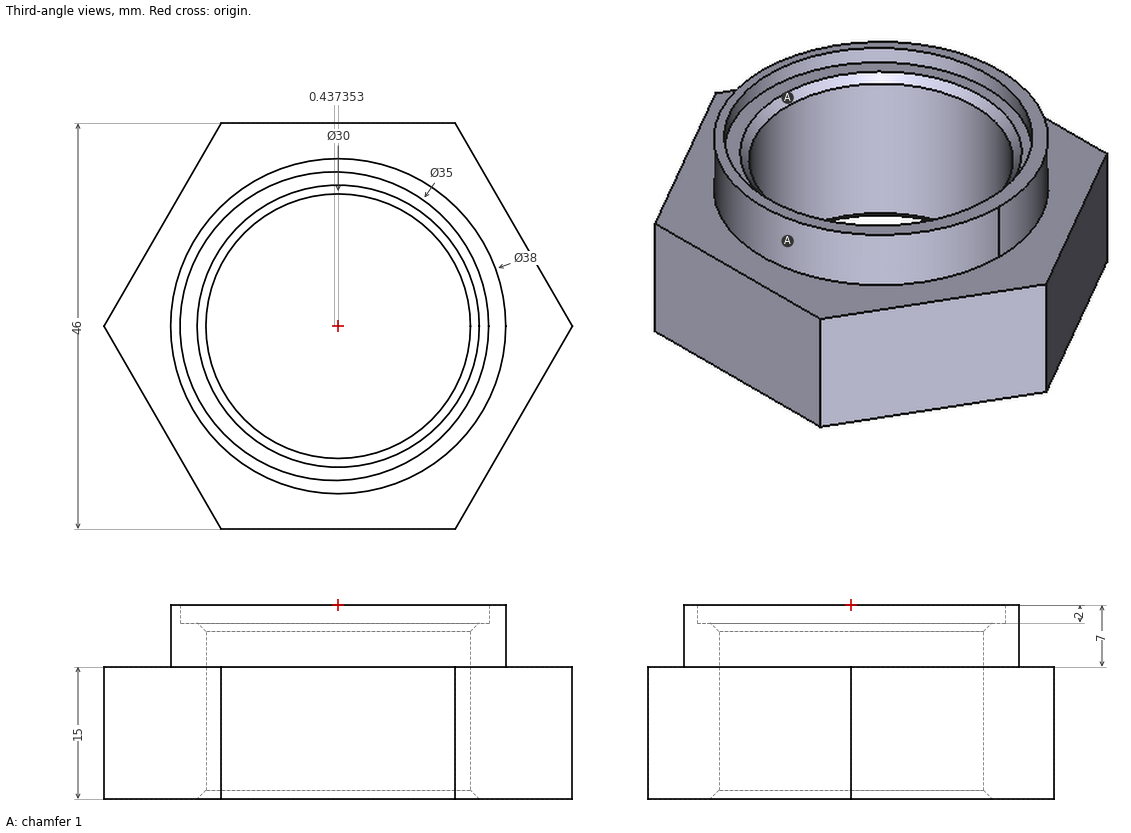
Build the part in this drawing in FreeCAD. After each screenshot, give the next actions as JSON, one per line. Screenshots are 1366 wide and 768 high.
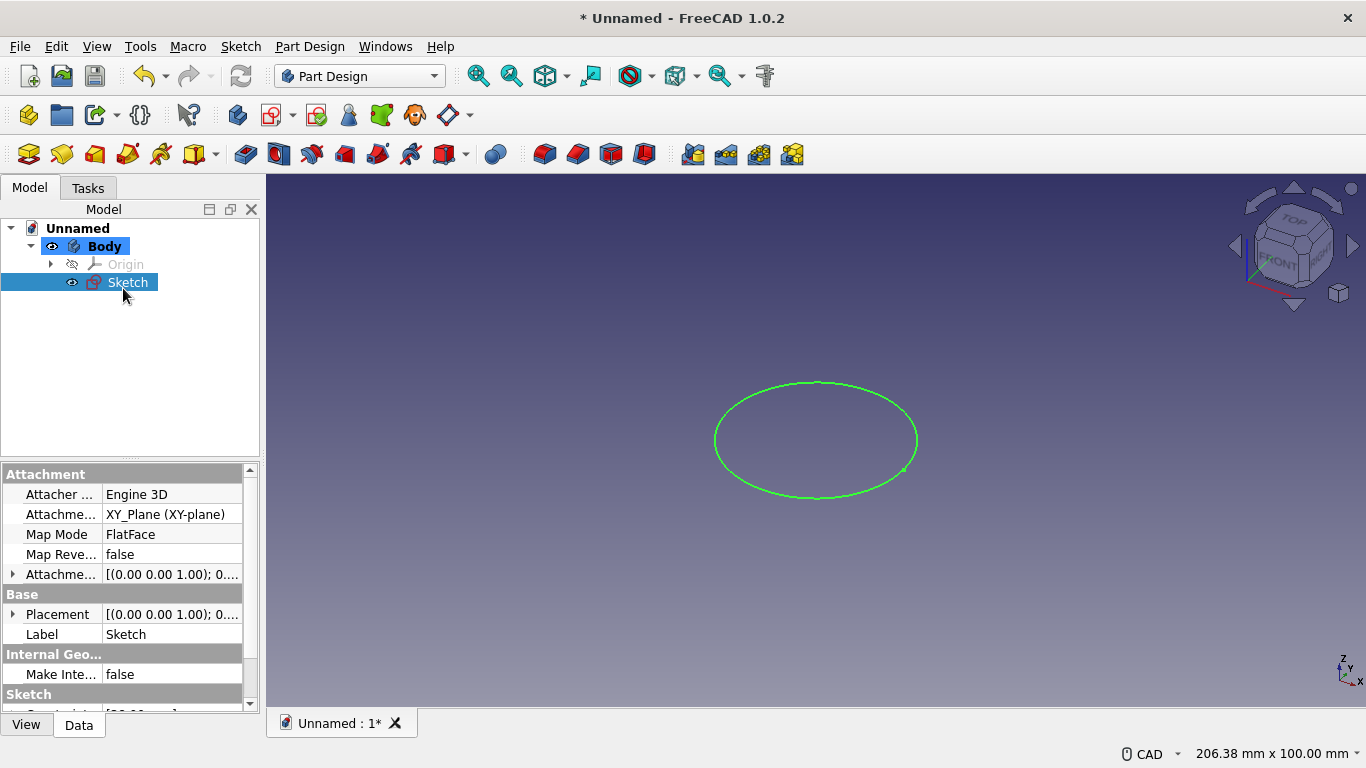
{"action": "left_click", "coordinate": [29, 154]}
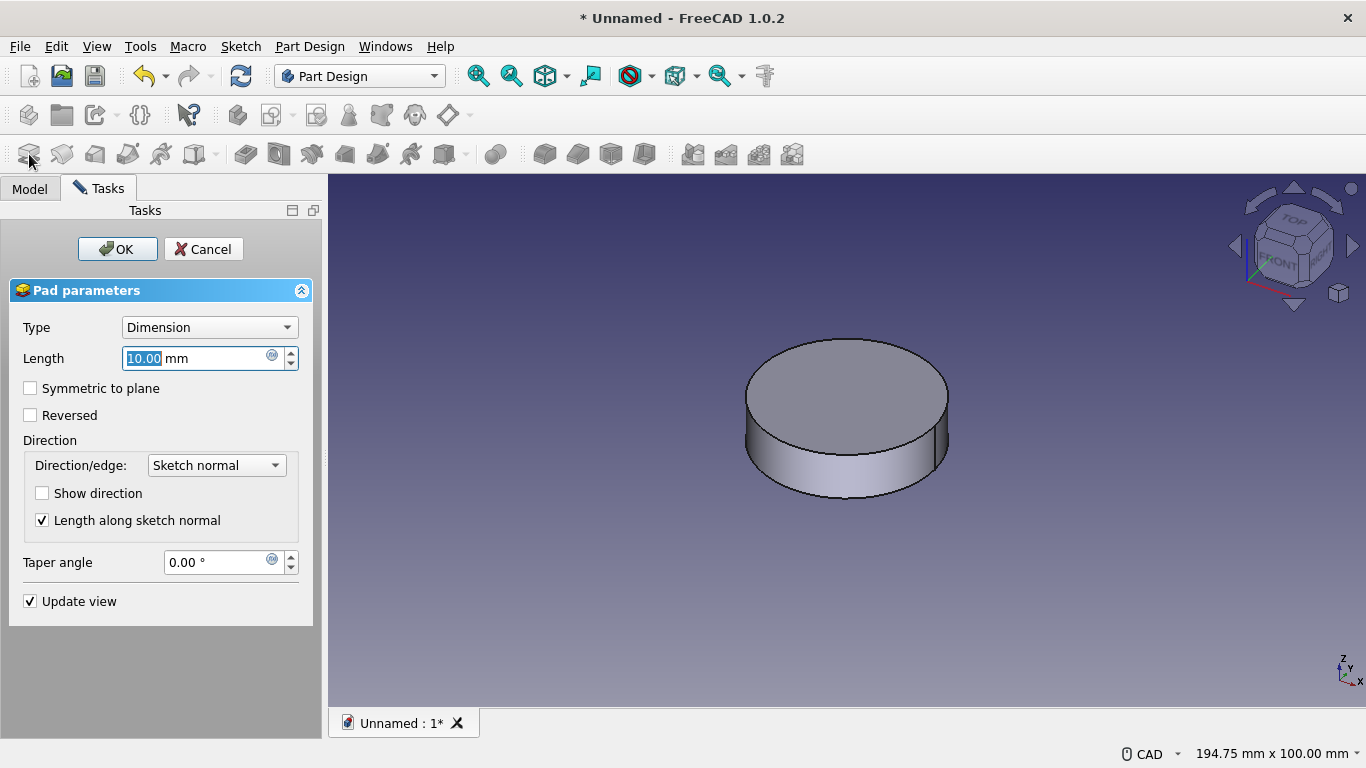
{"action": "type", "text": "7"}
{"action": "key", "text": "Tab"}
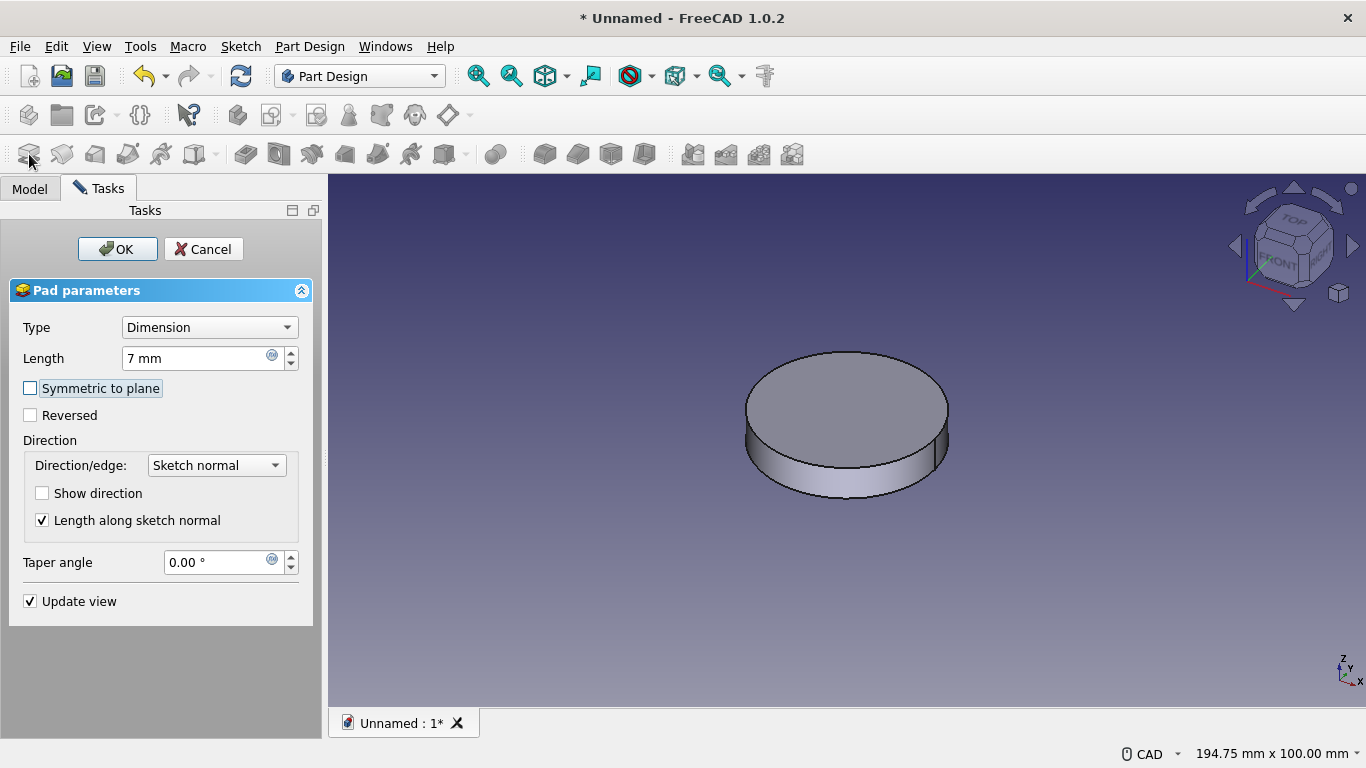
{"action": "left_click", "coordinate": [31, 415]}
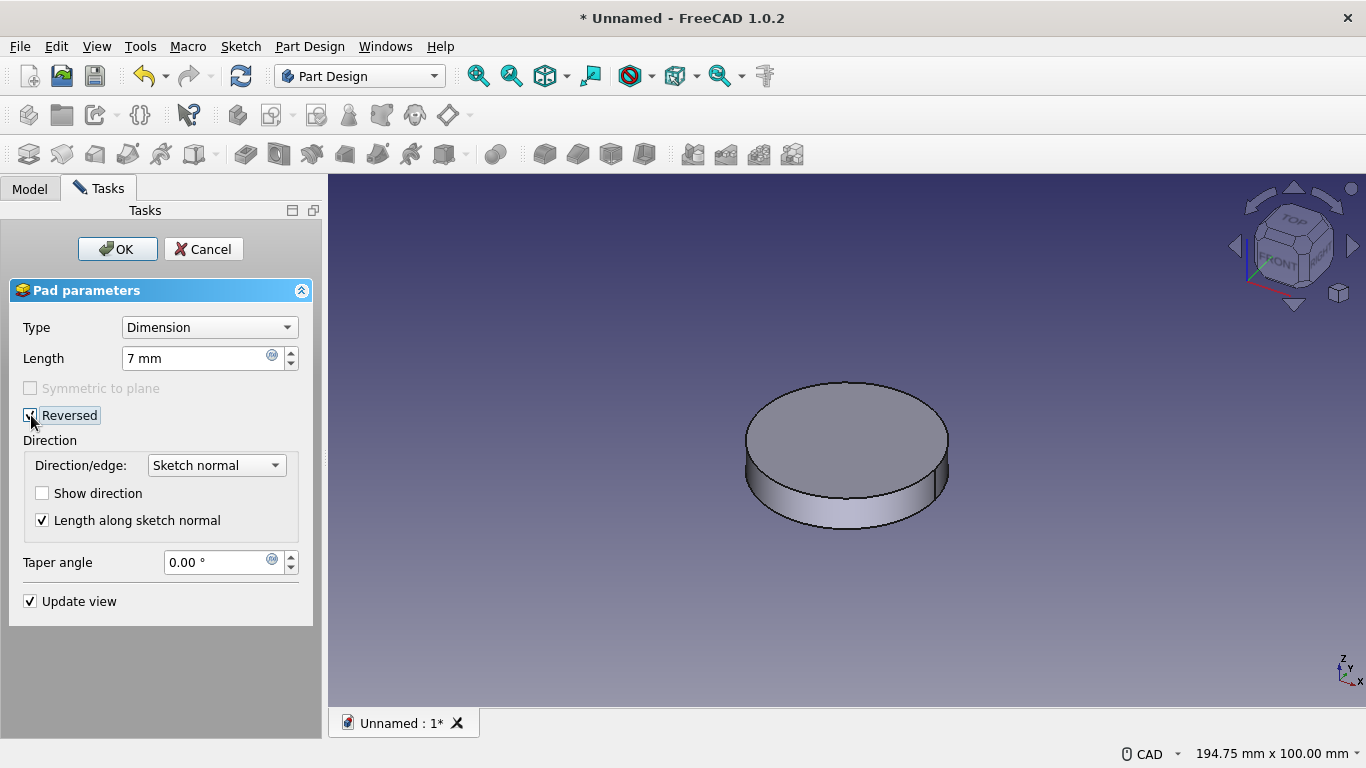
{"action": "left_click", "coordinate": [118, 249]}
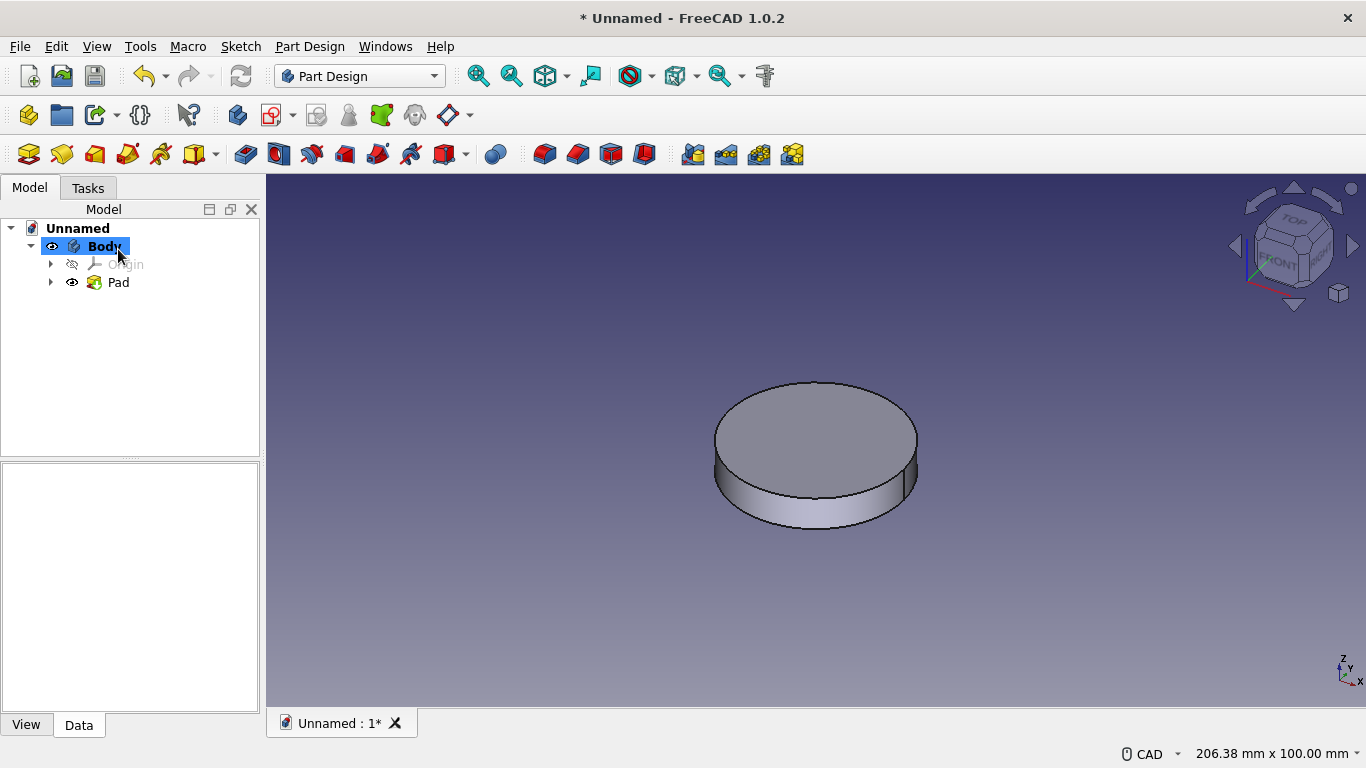
{"action": "left_click", "coordinate": [479, 76]}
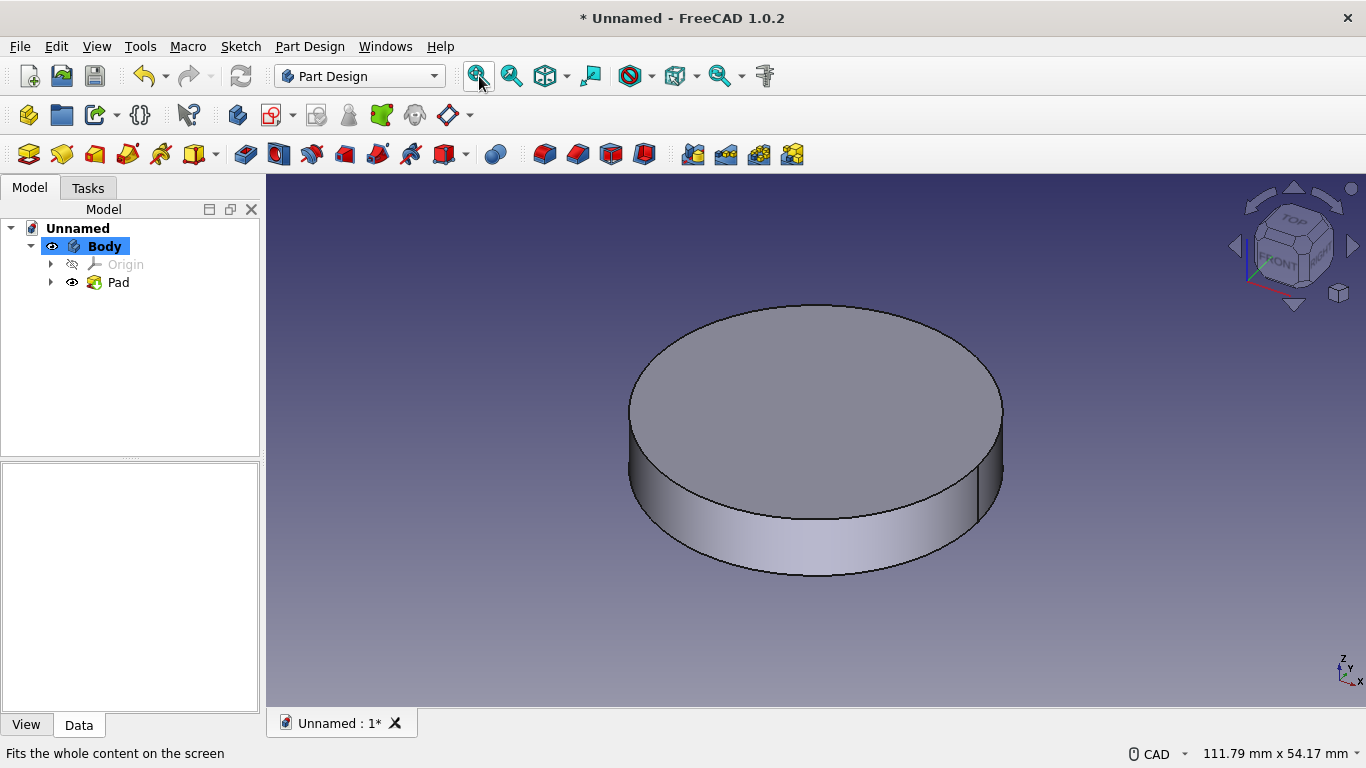
{"action": "key", "text": "5"}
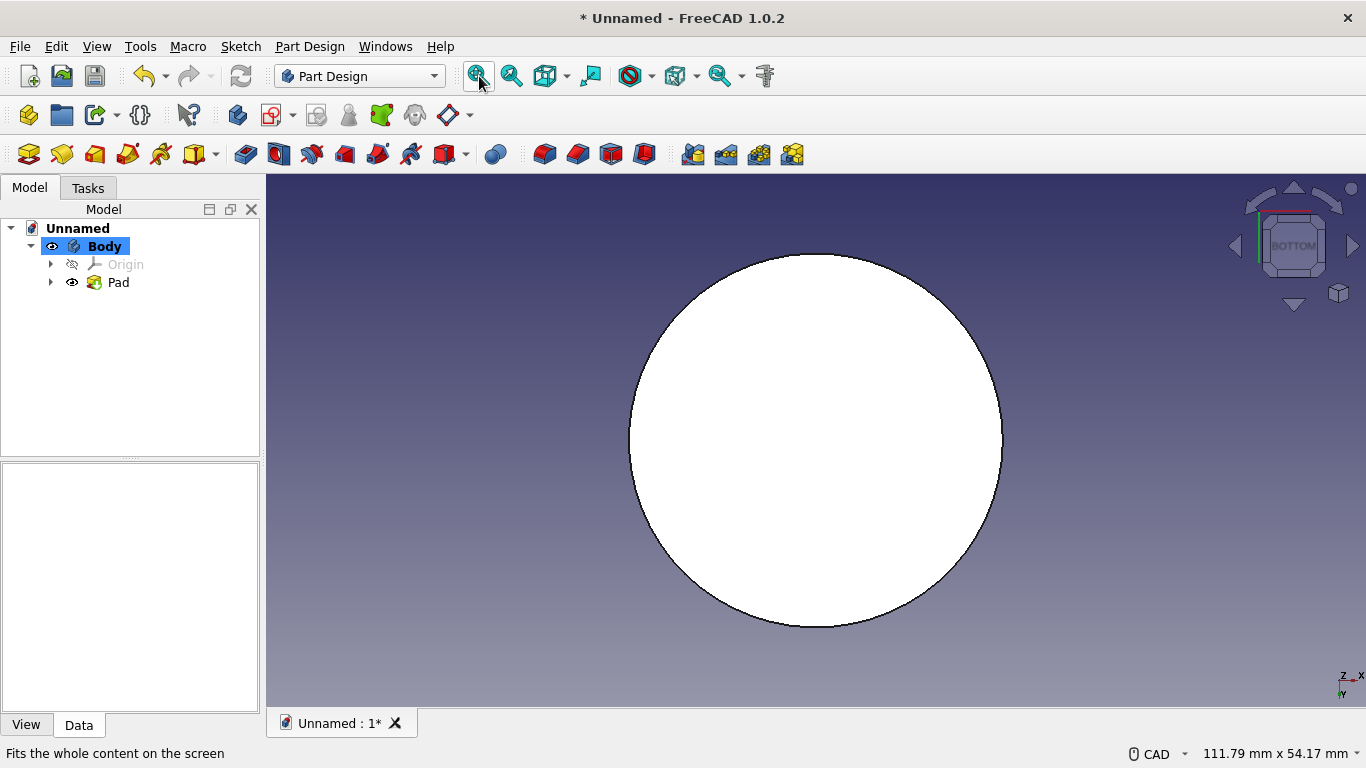
{"action": "left_click", "coordinate": [816, 439]}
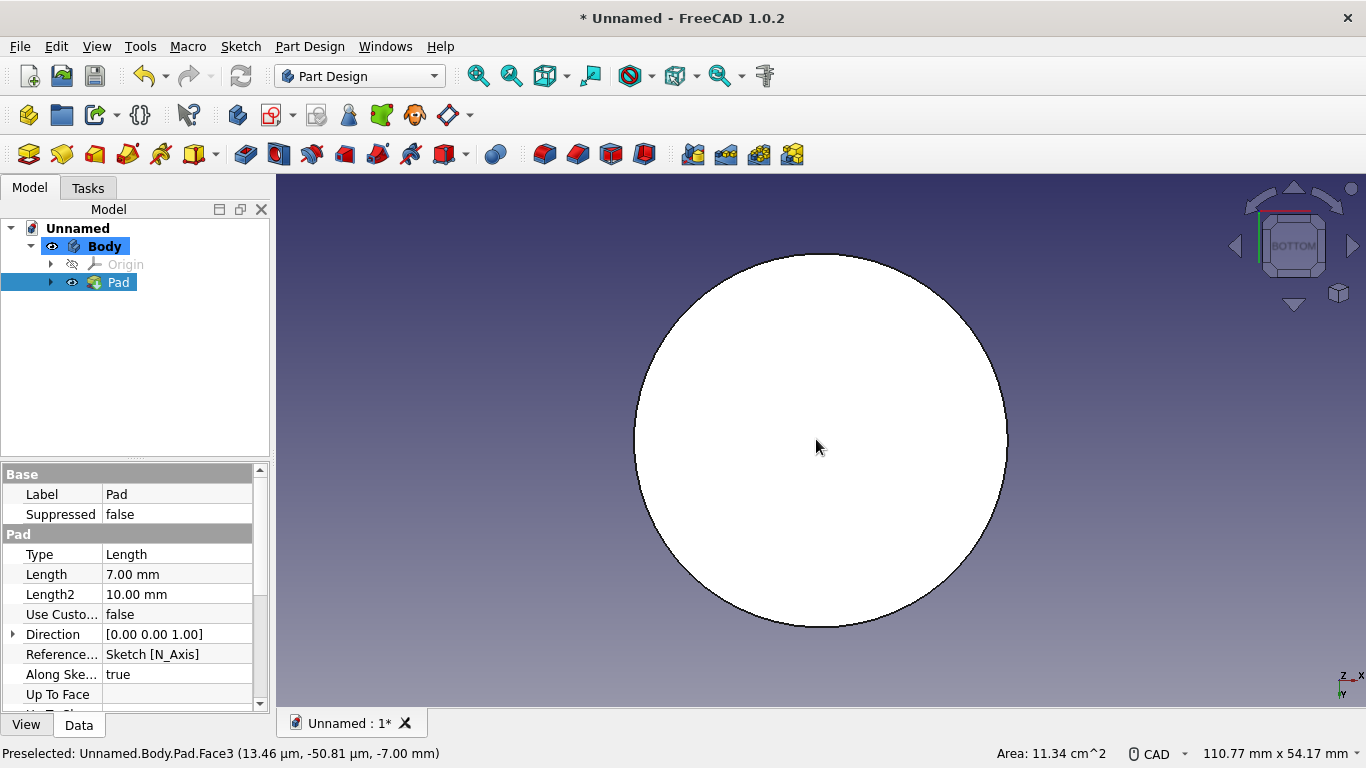
{"action": "left_click", "coordinate": [270, 116]}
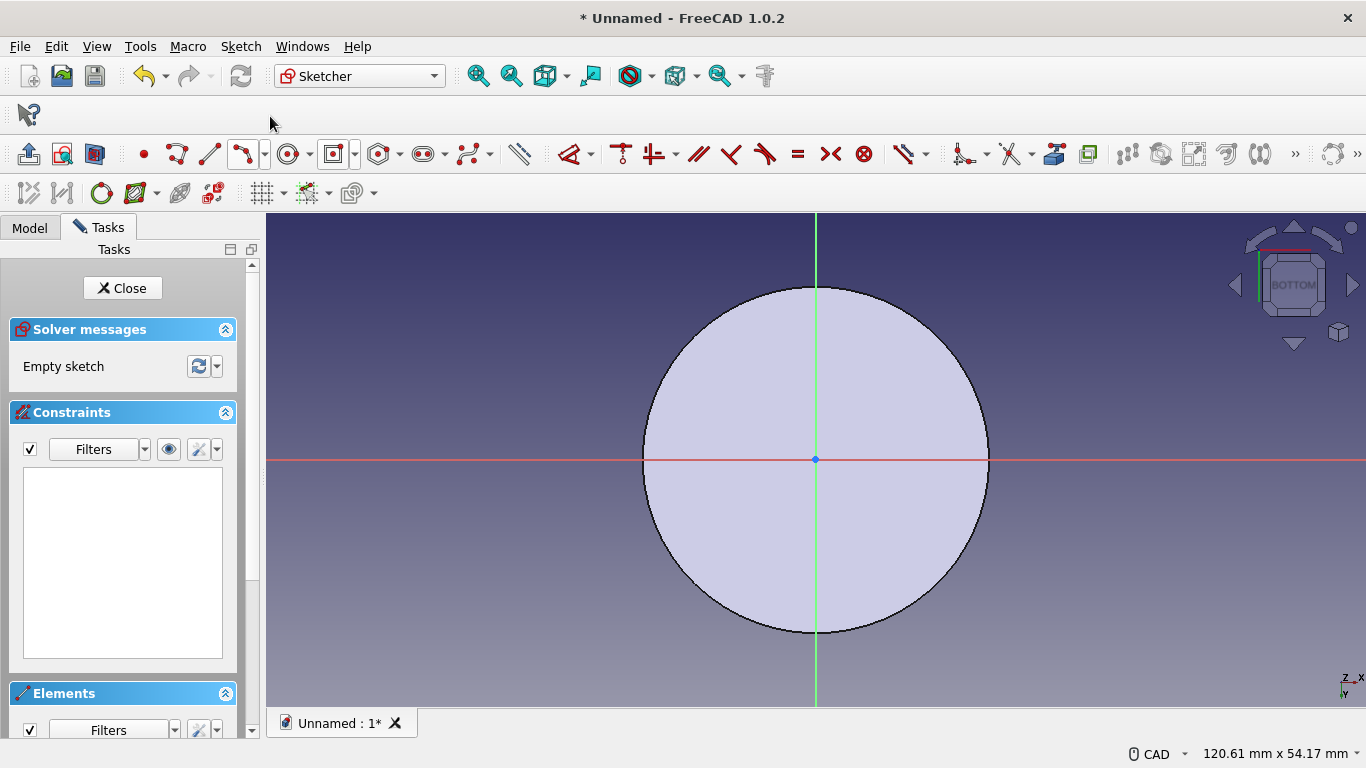
{"action": "scroll", "coordinate": [608, 460], "scroll_direction": "down", "scroll_amount": 2}